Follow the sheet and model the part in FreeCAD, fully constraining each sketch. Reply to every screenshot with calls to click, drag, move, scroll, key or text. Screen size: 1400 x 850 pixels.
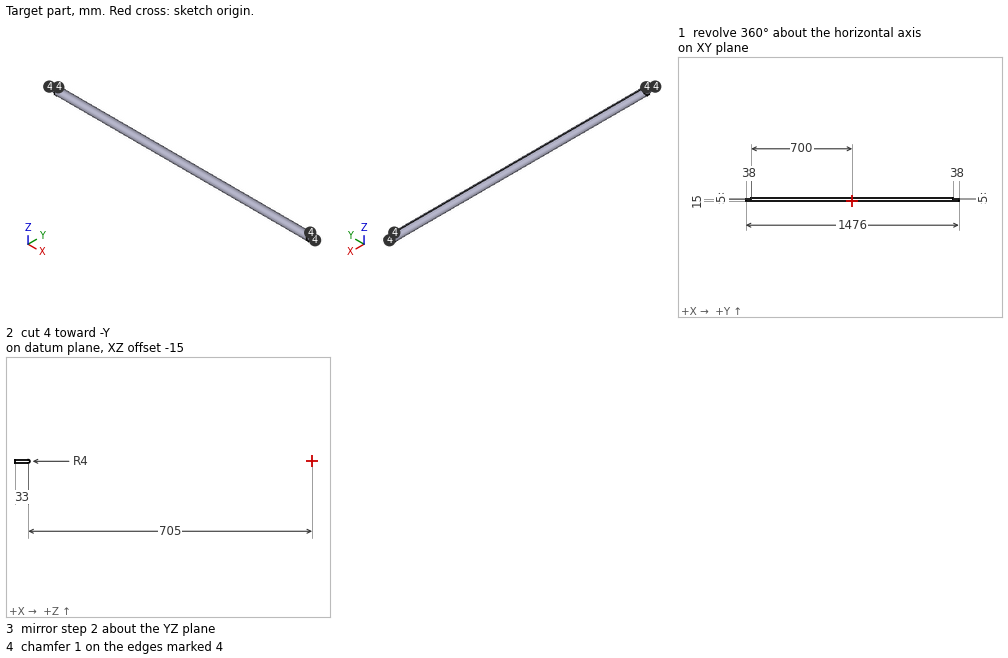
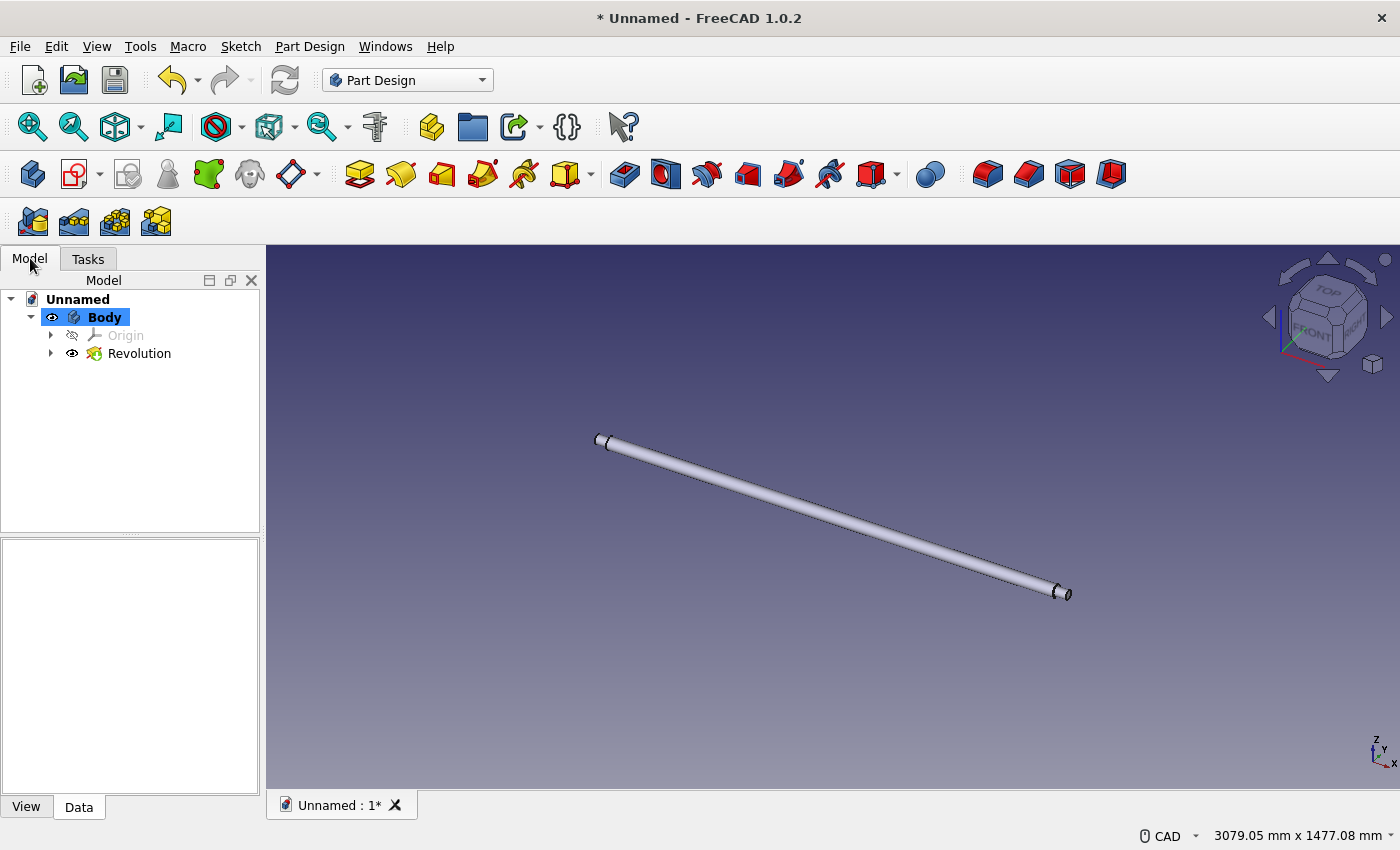
click(51, 335)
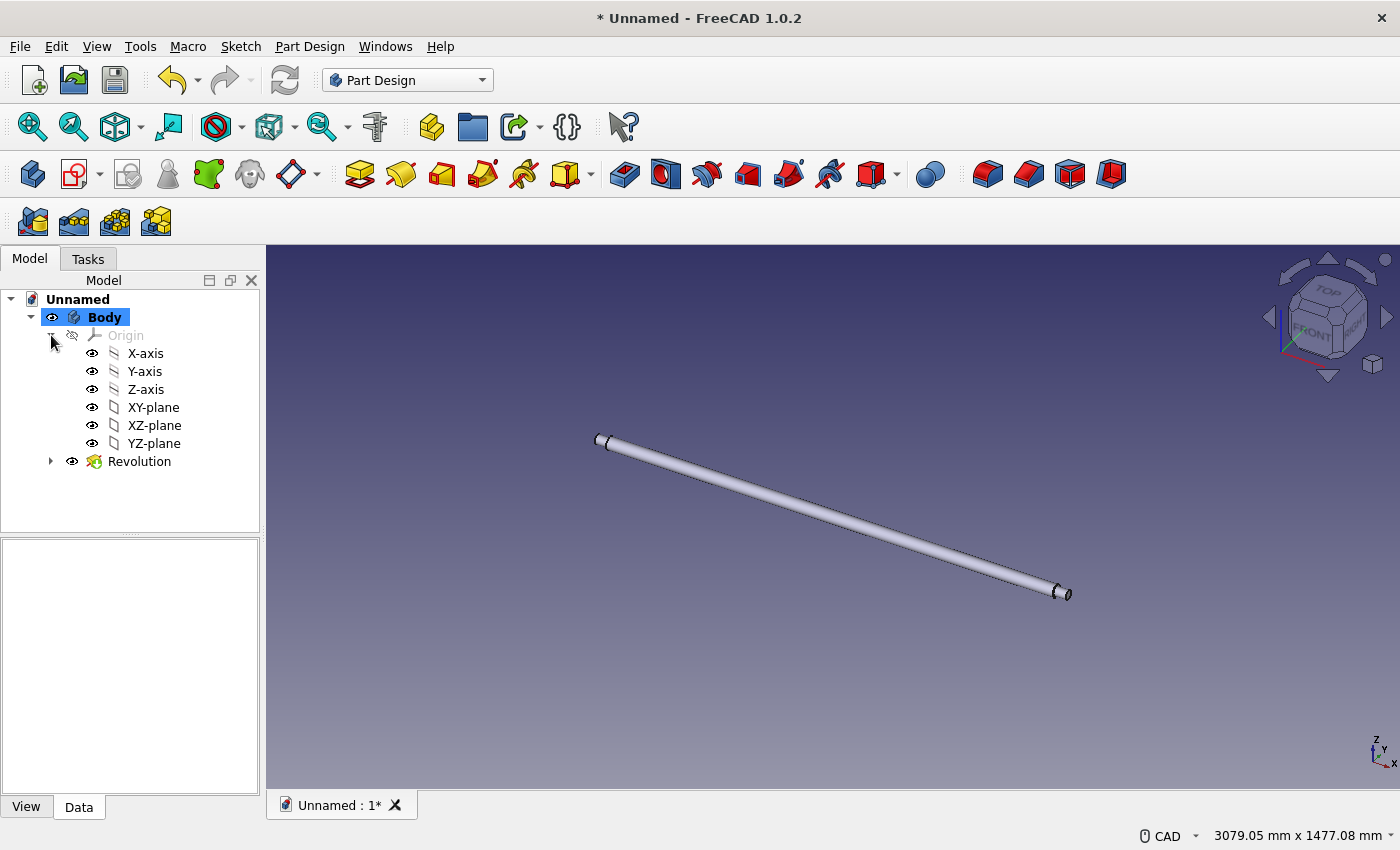
click(137, 425)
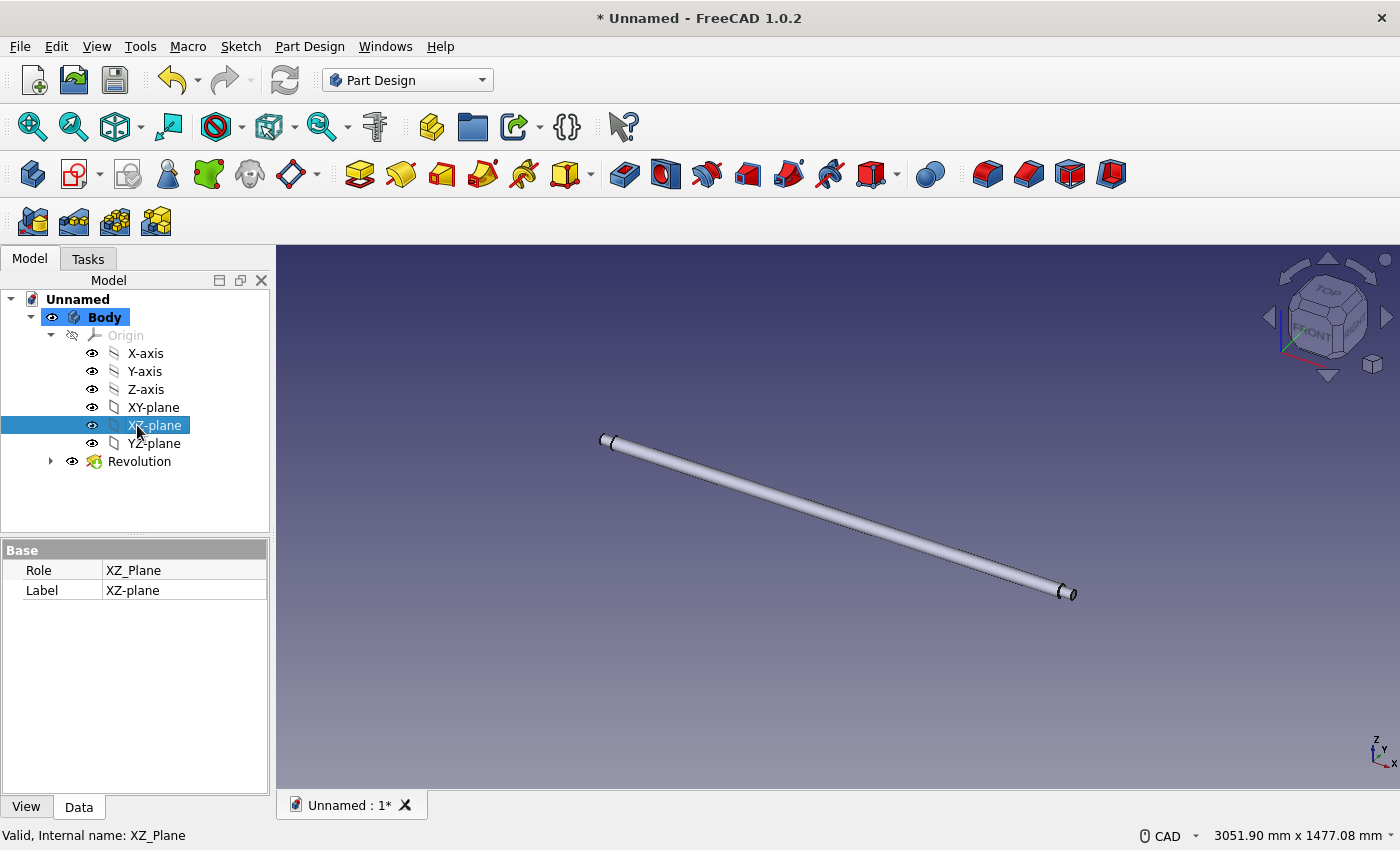
click(290, 174)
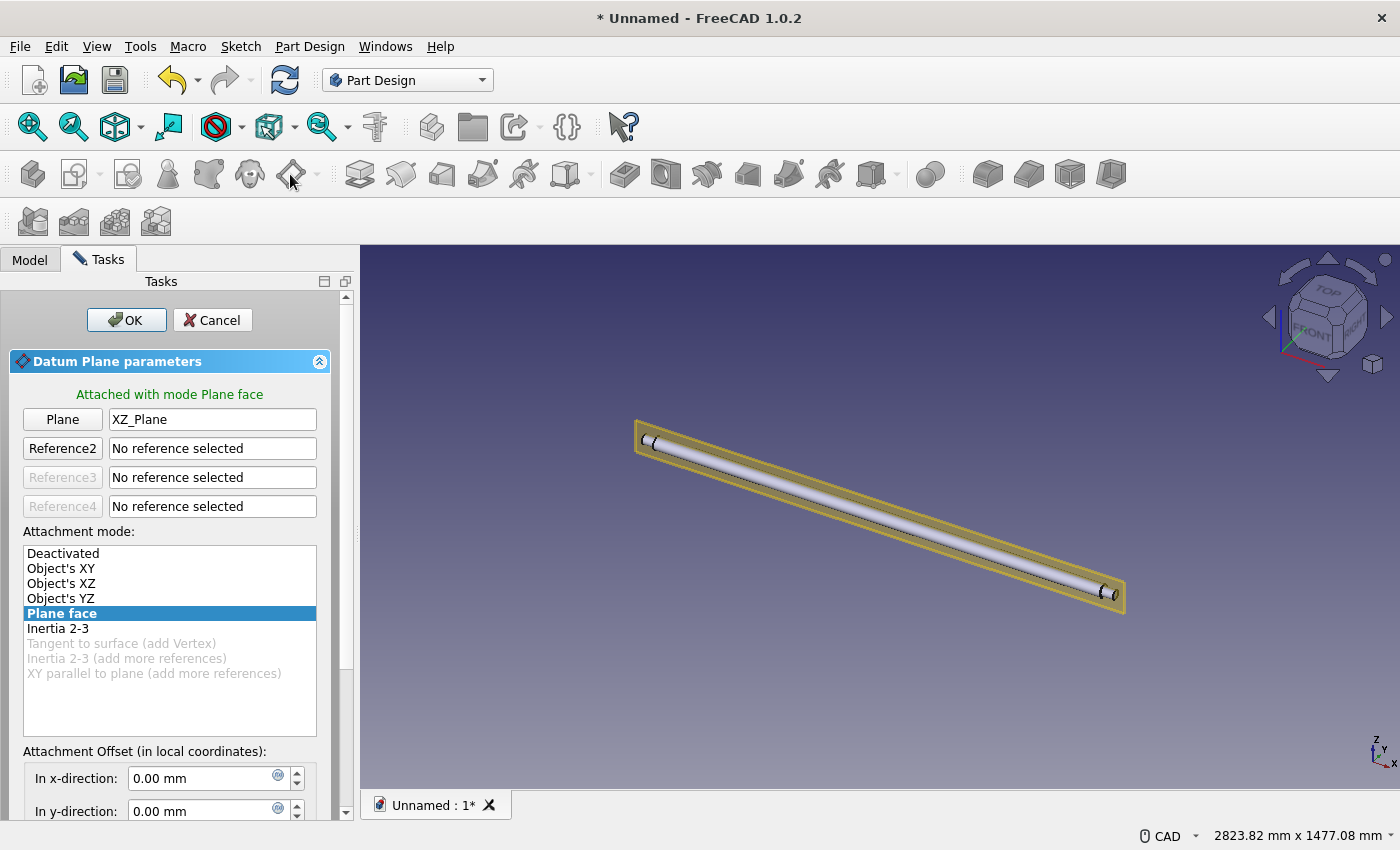
scroll(346, 556, down, 2)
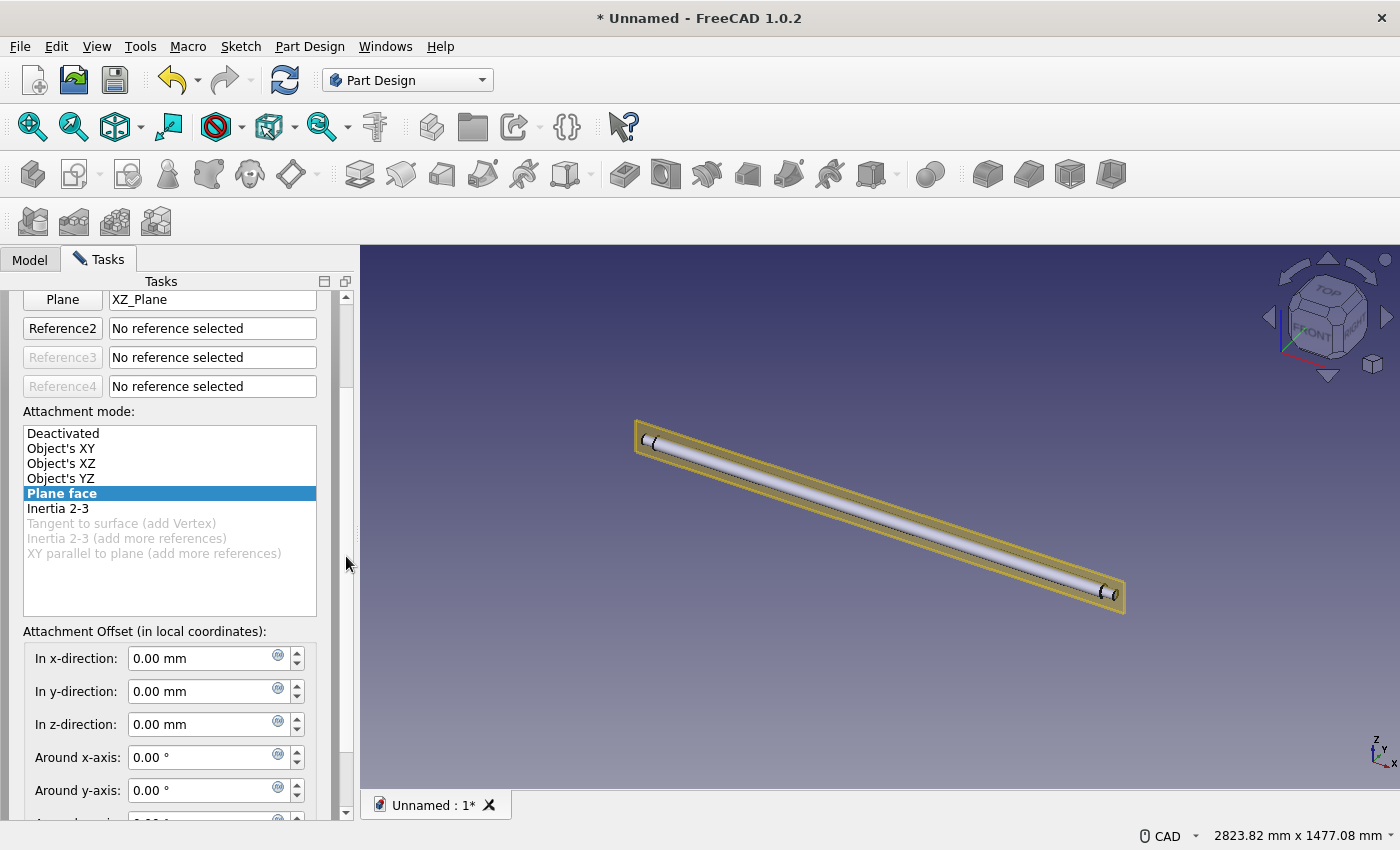
triple_click(210, 724)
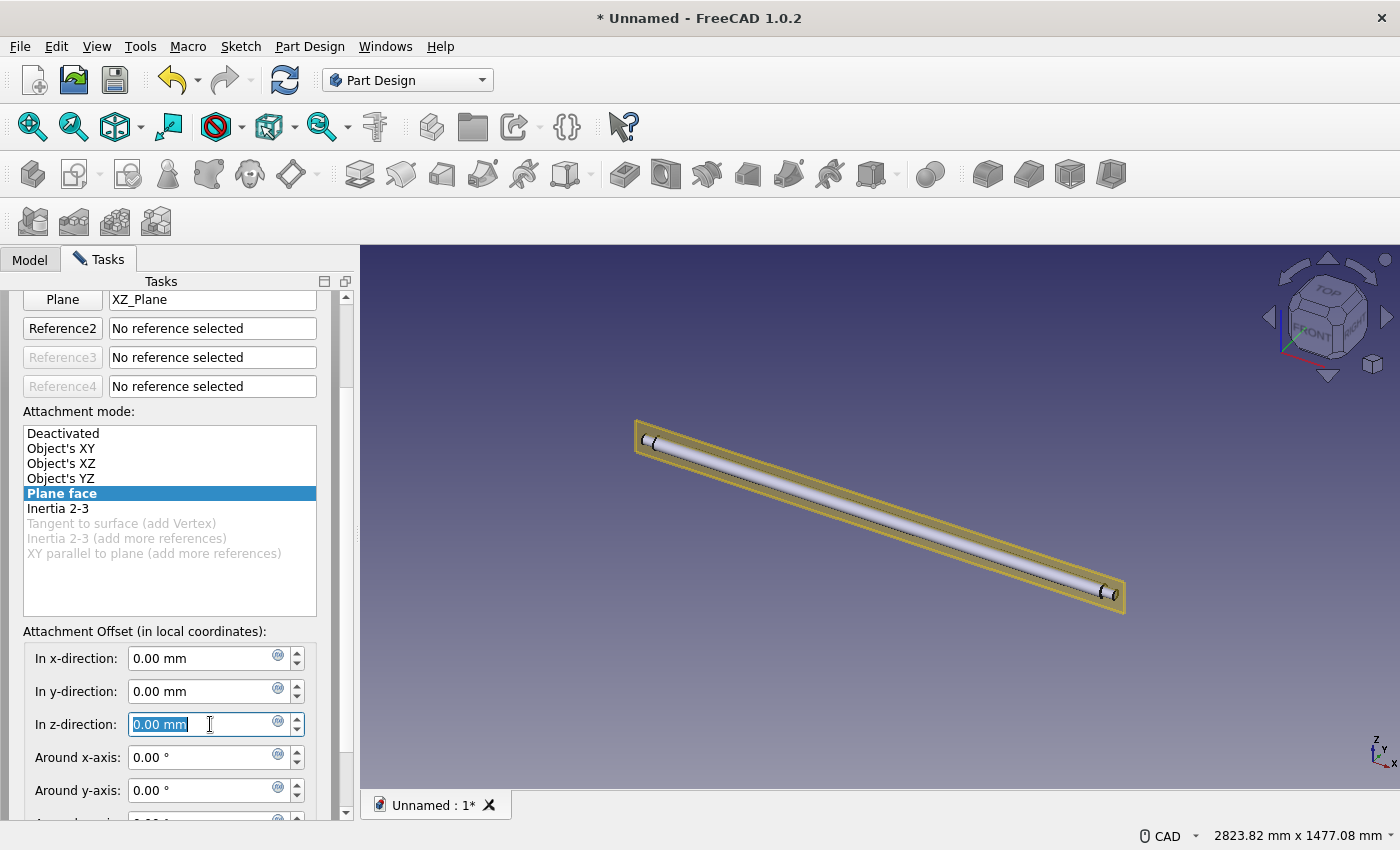
text(-15)
key(Tab)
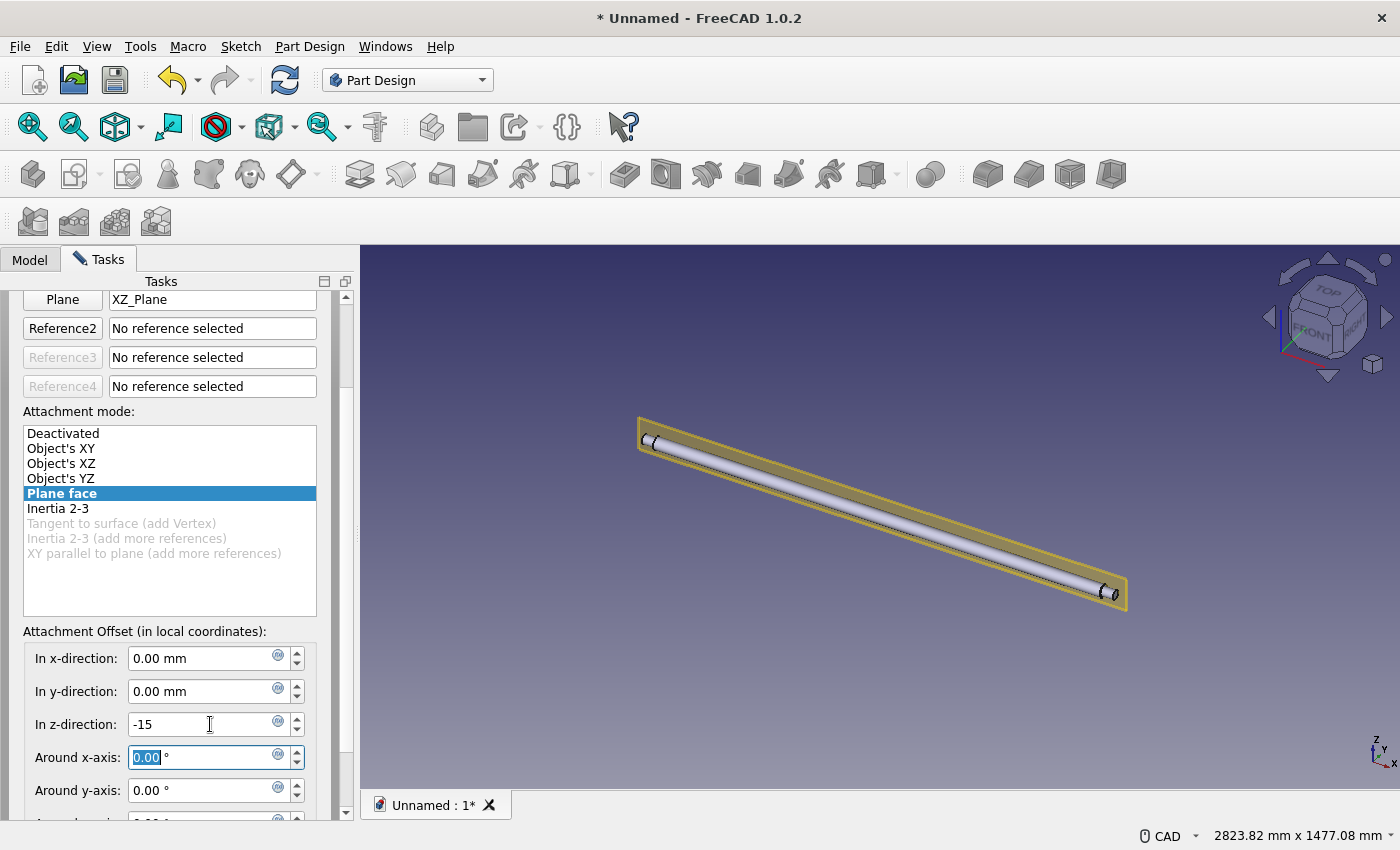
scroll(346, 556, up, 3)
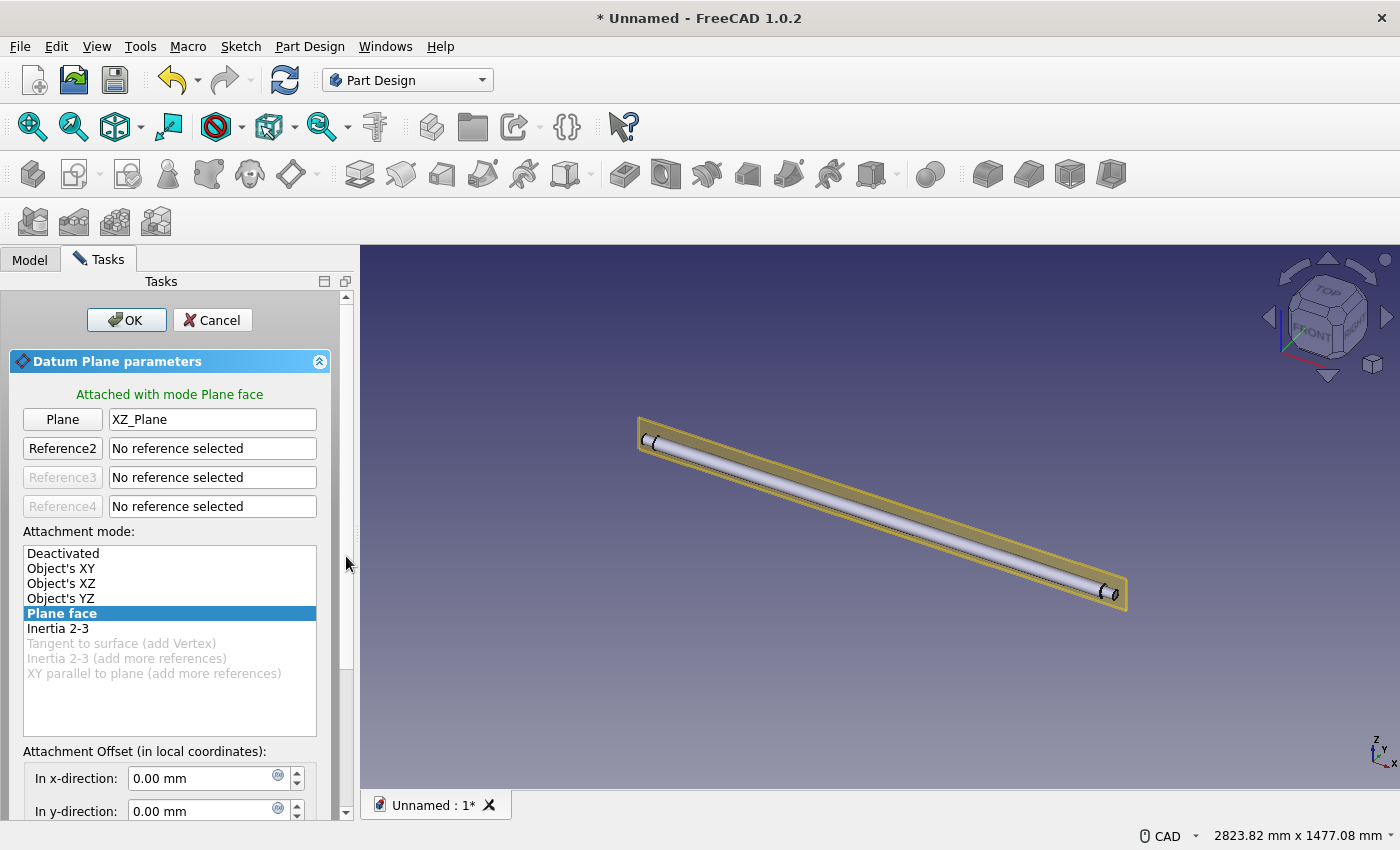
click(127, 320)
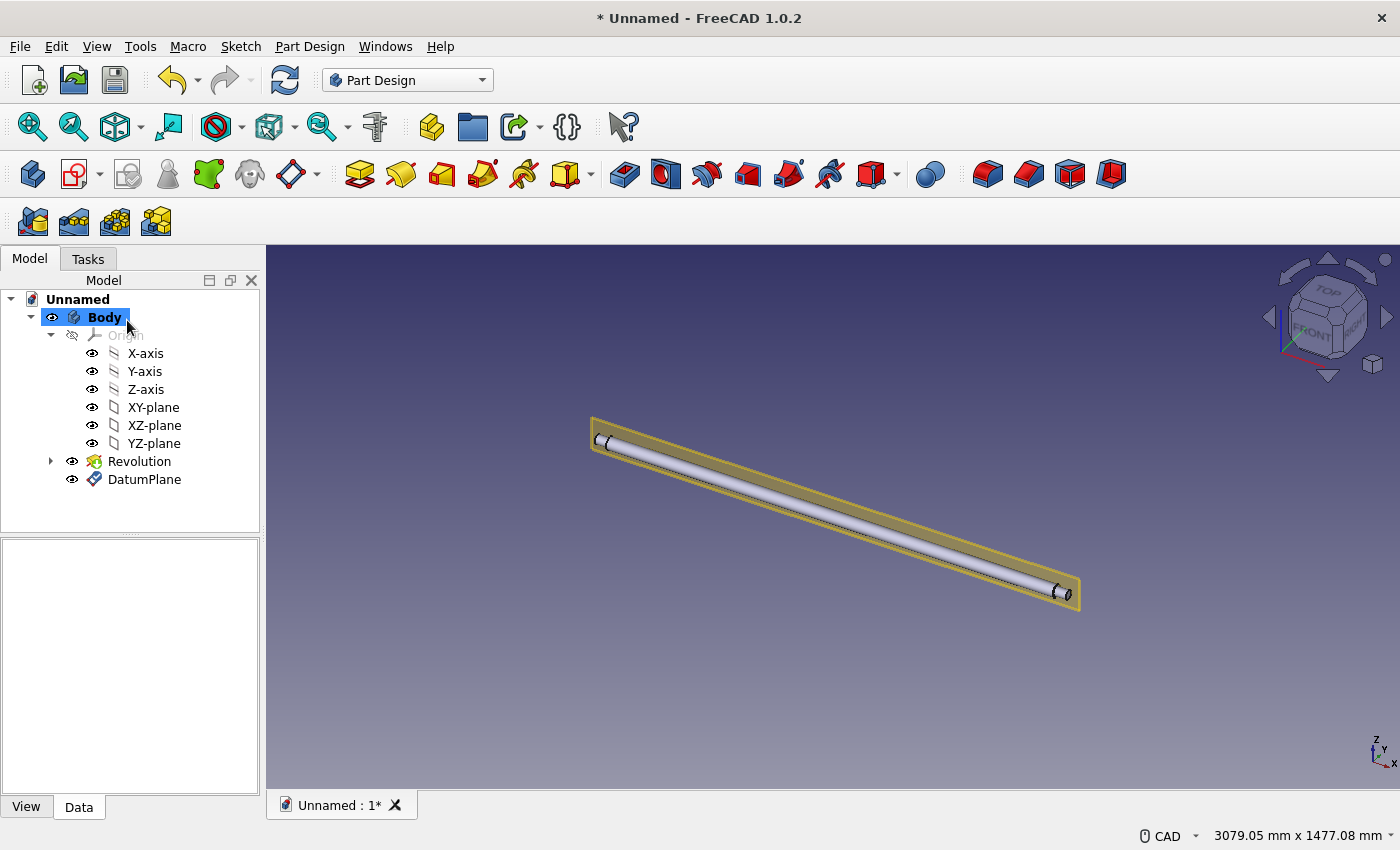
click(117, 479)